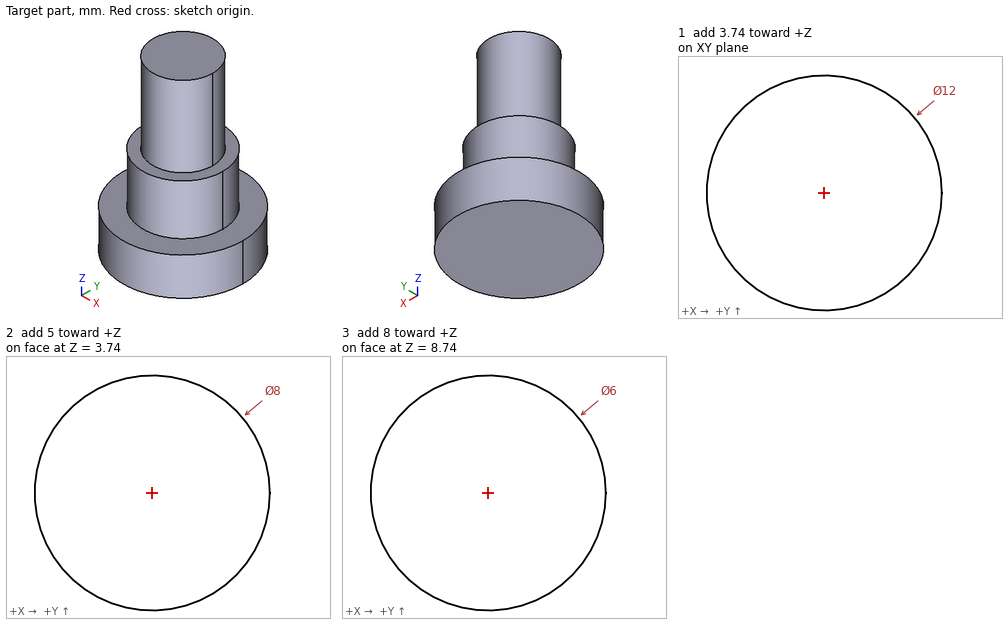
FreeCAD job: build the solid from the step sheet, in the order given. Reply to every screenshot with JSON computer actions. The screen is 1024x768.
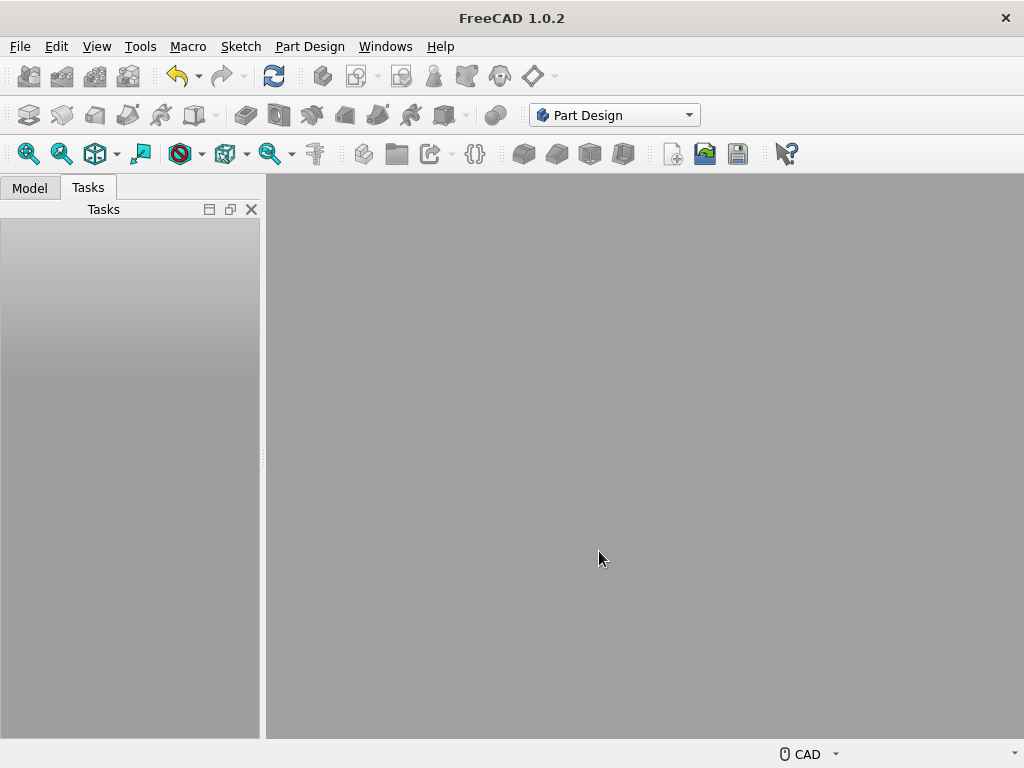
{"action": "key", "text": "ctrl+n"}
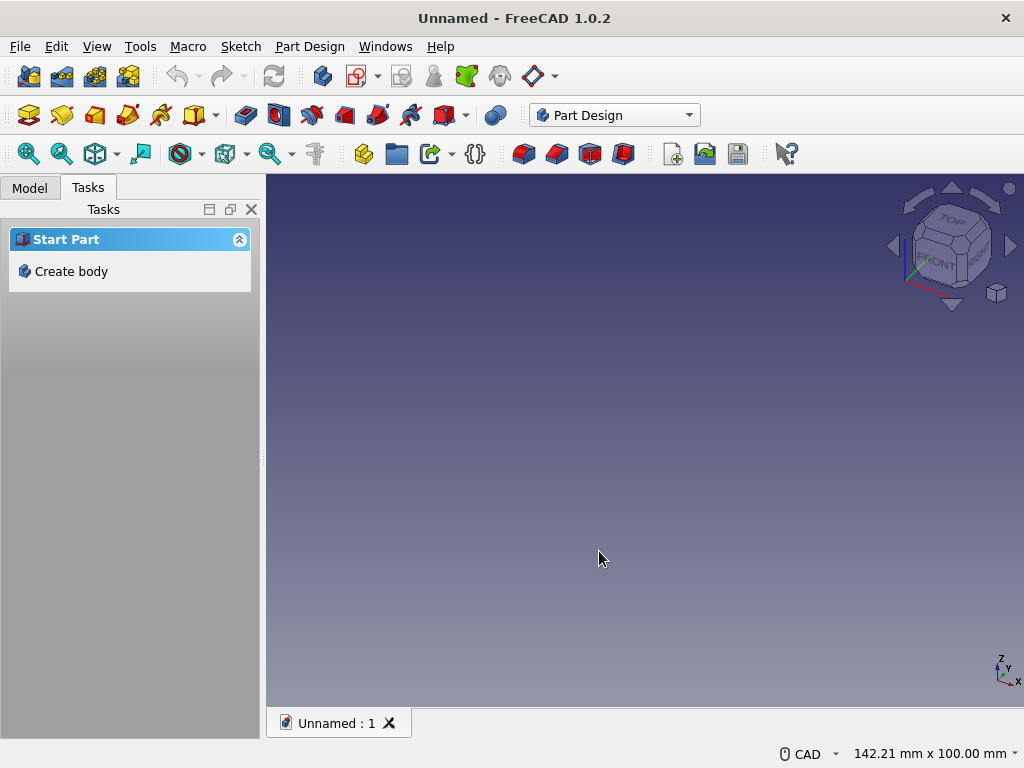
{"action": "left_click", "coordinate": [356, 76]}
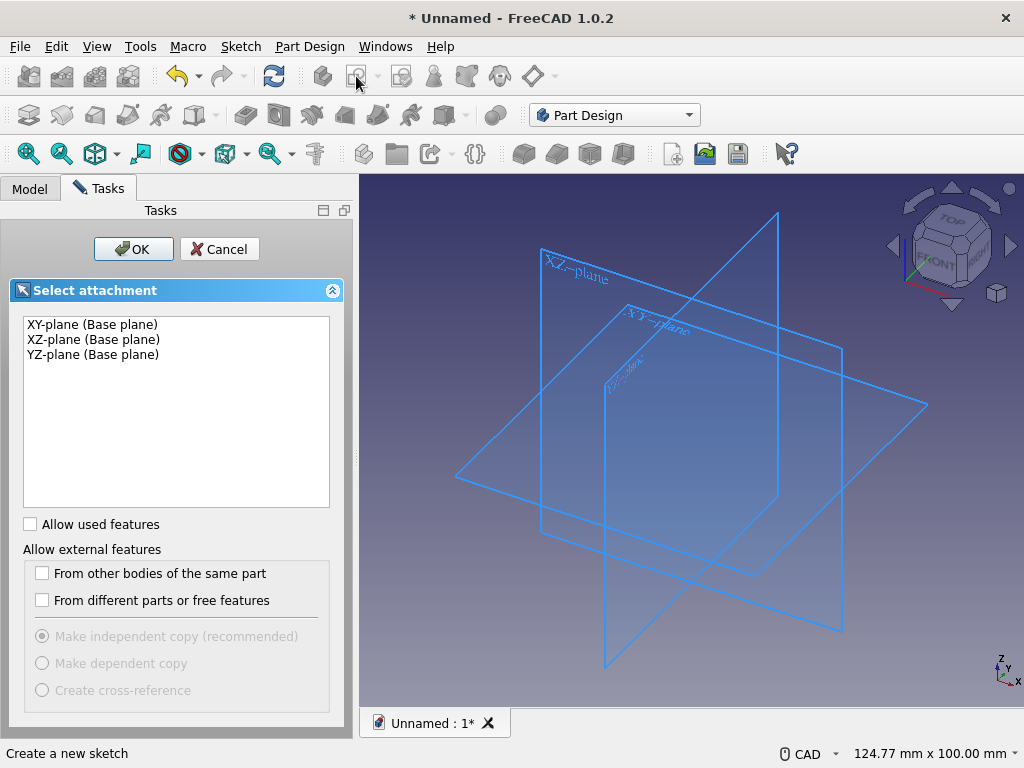
{"action": "left_click", "coordinate": [84, 324]}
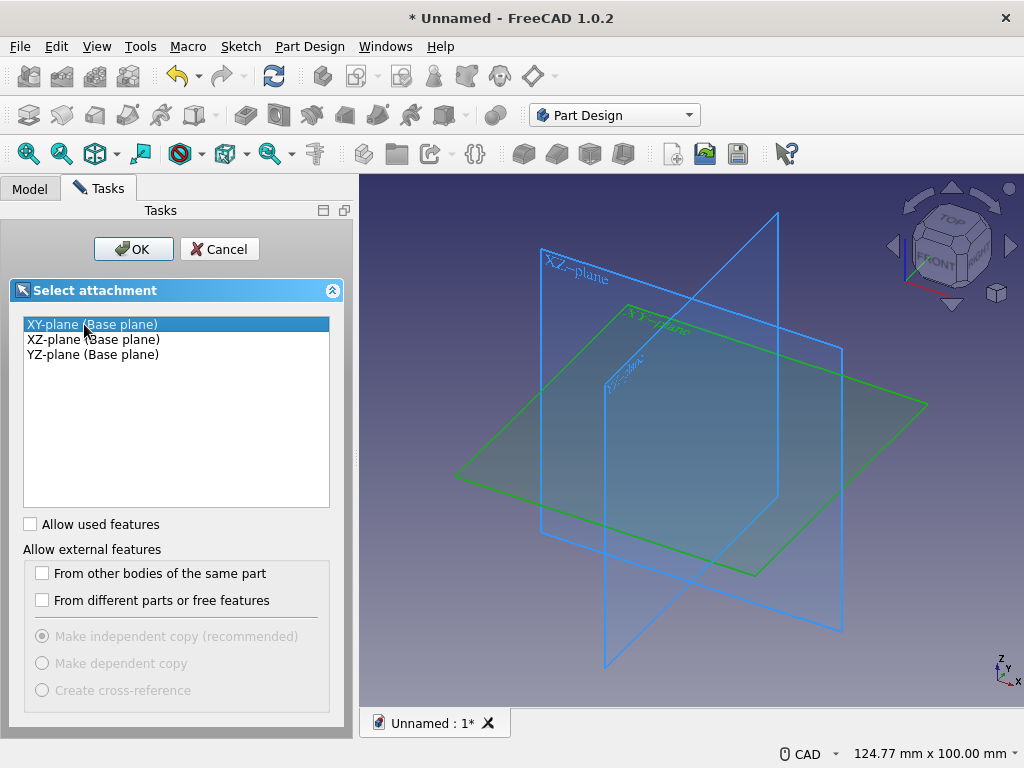
{"action": "left_click", "coordinate": [134, 249]}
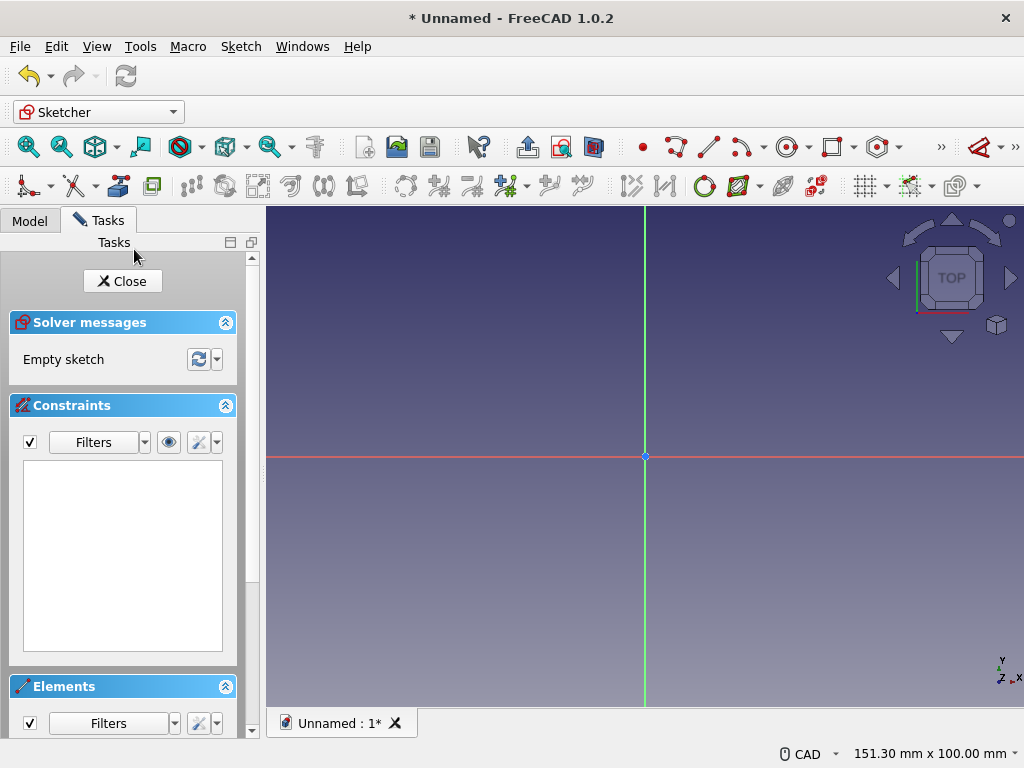
{"action": "scroll", "coordinate": [662, 456], "scroll_direction": "up", "scroll_amount": 8}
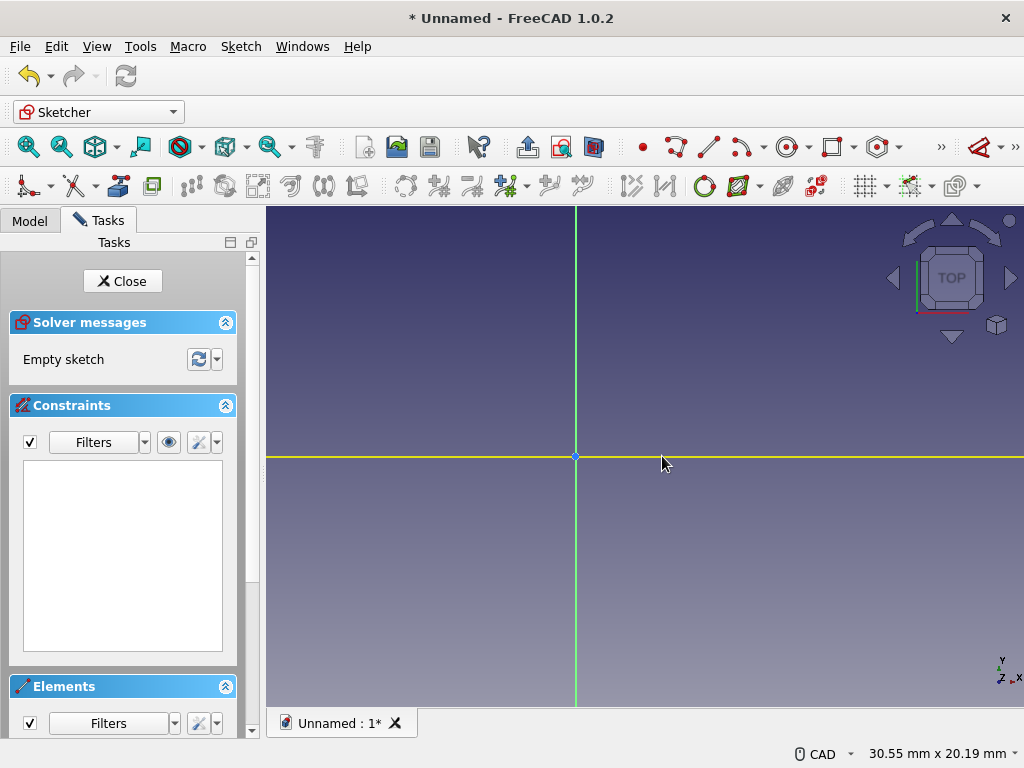
{"action": "left_click", "coordinate": [786, 148]}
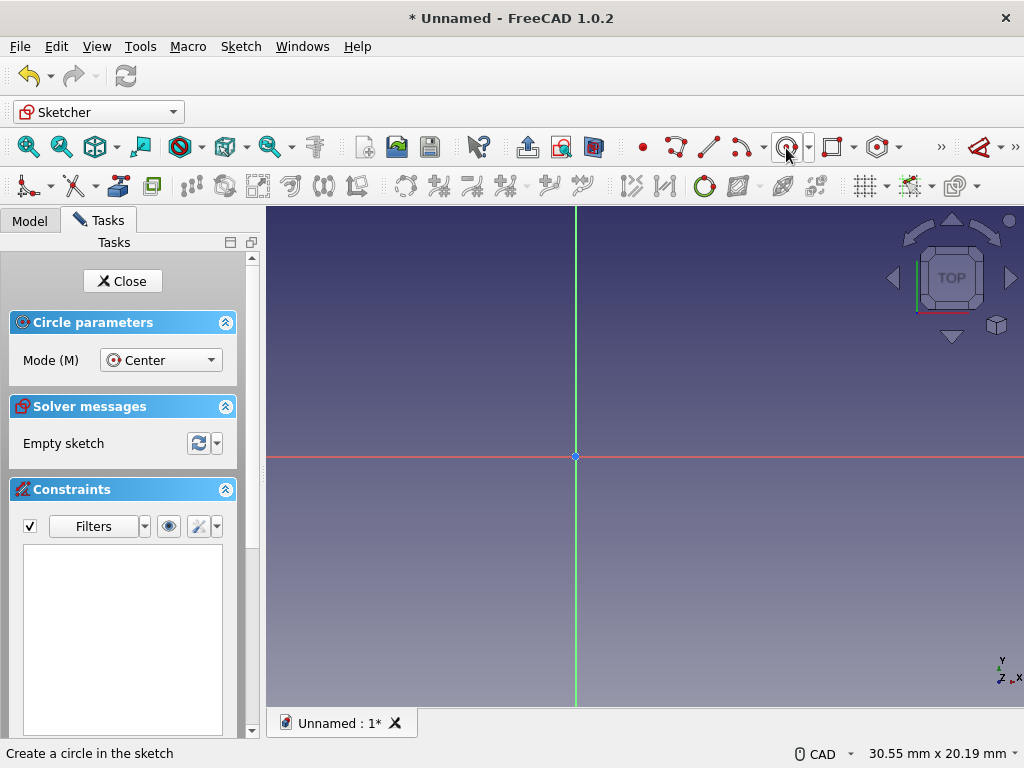
{"action": "left_click", "coordinate": [576, 456]}
{"action": "left_click", "coordinate": [681, 351]}
{"action": "key", "text": "Escape"}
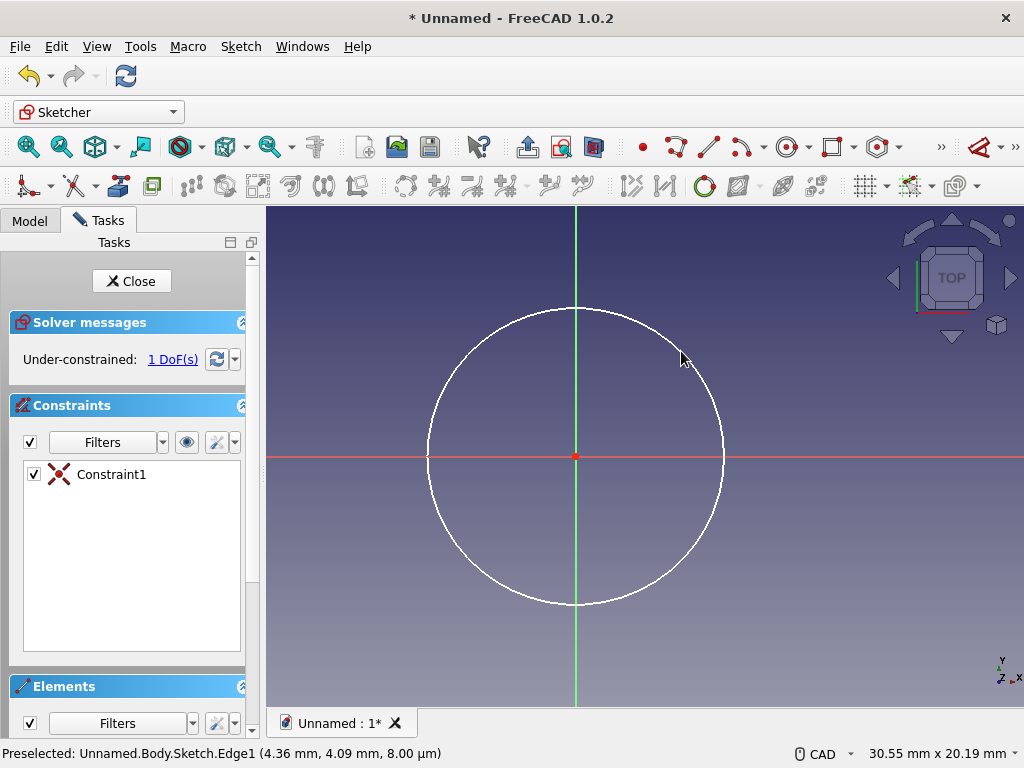
{"action": "left_click", "coordinate": [680, 351]}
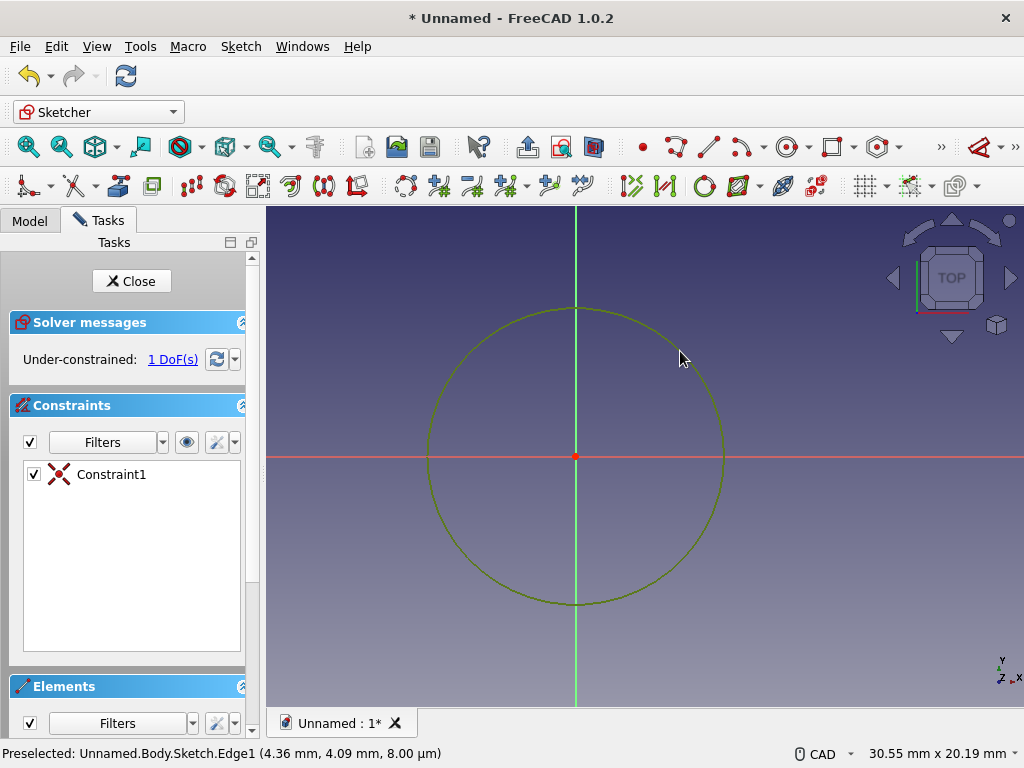
{"action": "left_click", "coordinate": [1000, 148]}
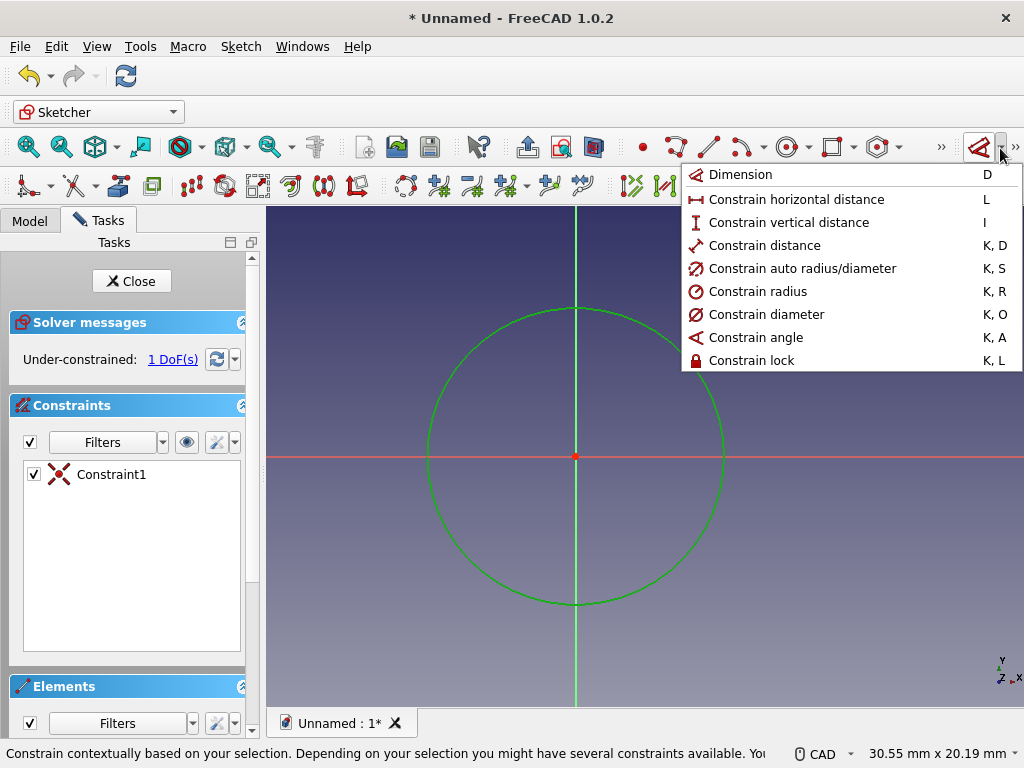
{"action": "left_click", "coordinate": [852, 314]}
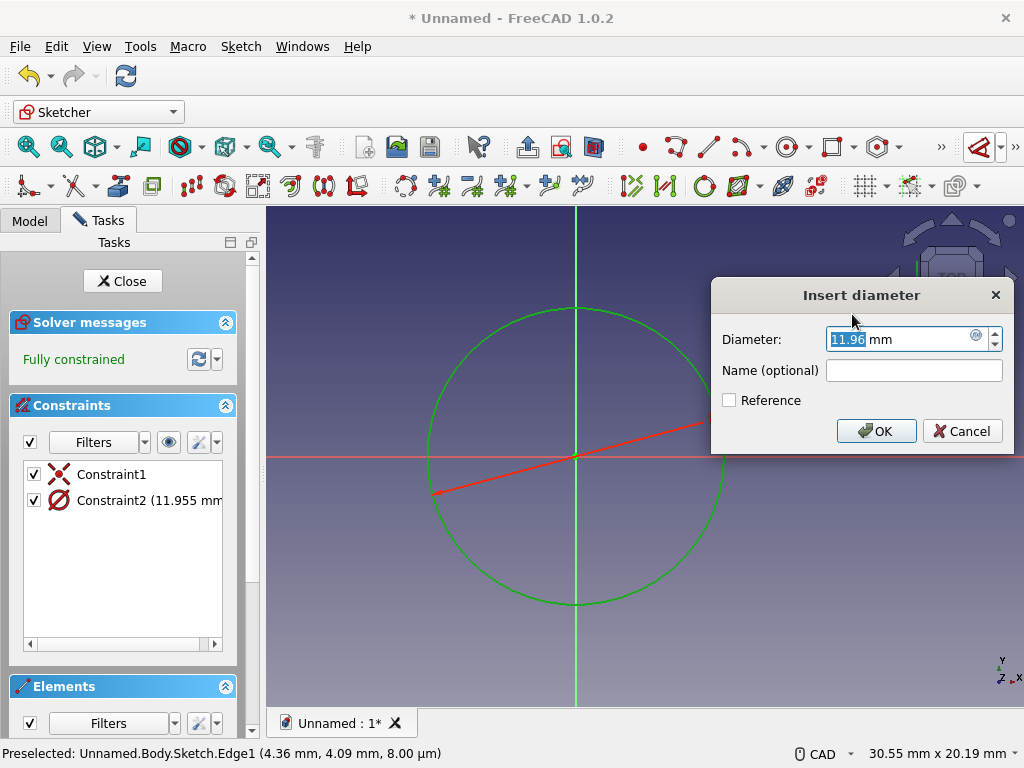
{"action": "type", "text": "12"}
{"action": "key", "text": "Return"}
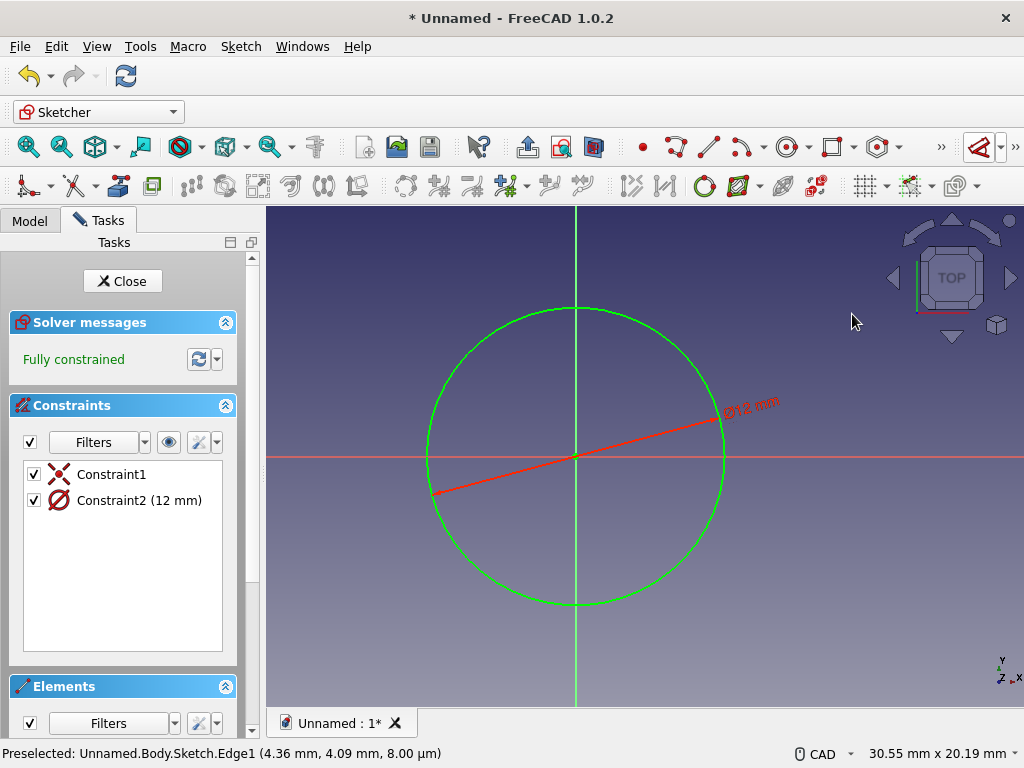
{"action": "left_click", "coordinate": [123, 281]}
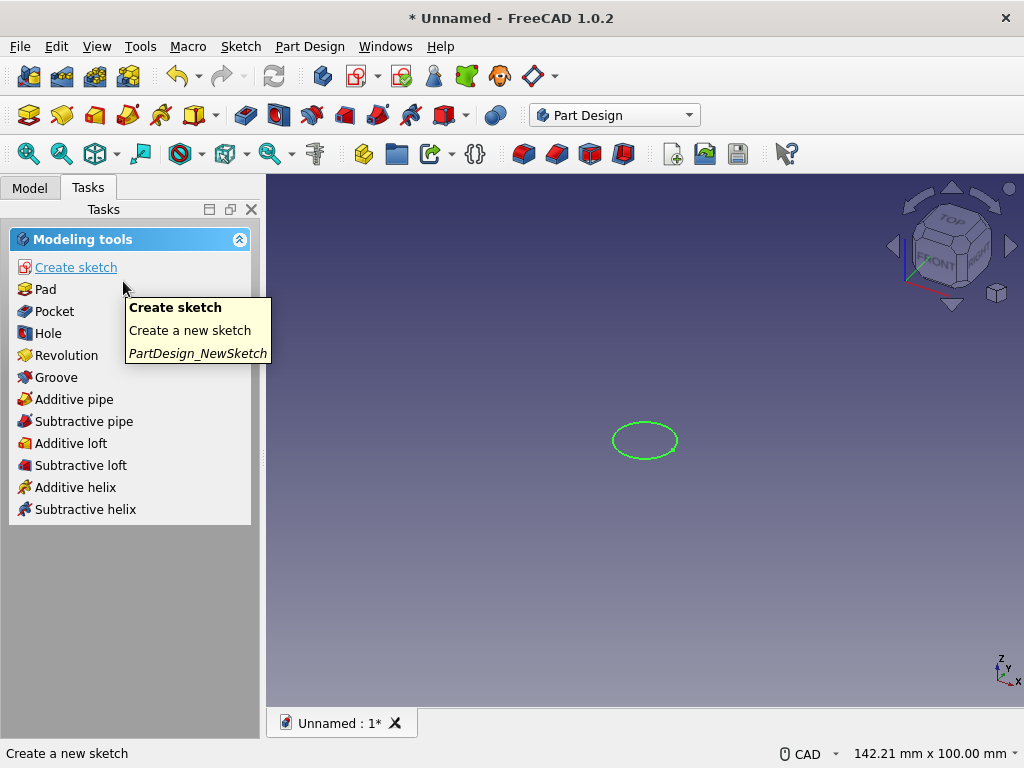
{"action": "left_click", "coordinate": [29, 116]}